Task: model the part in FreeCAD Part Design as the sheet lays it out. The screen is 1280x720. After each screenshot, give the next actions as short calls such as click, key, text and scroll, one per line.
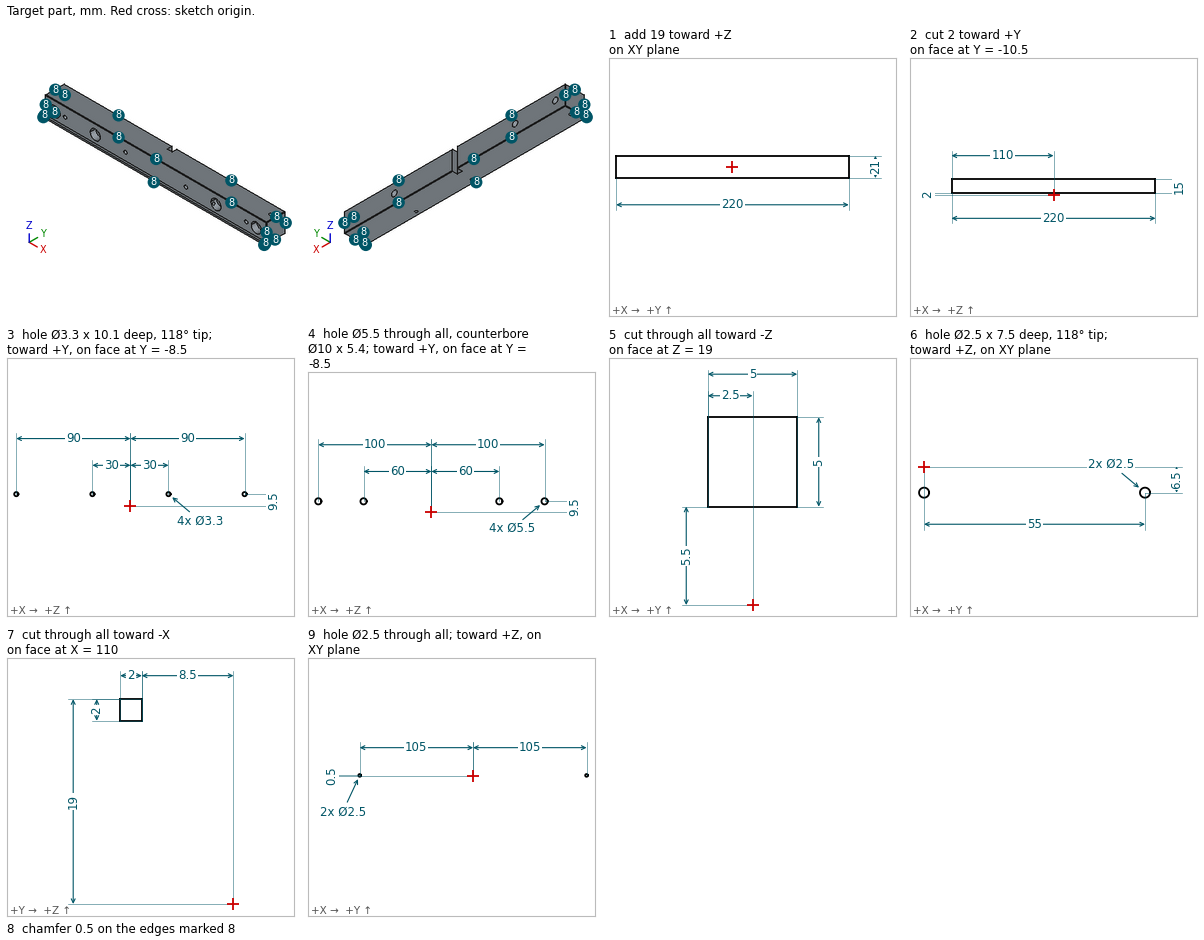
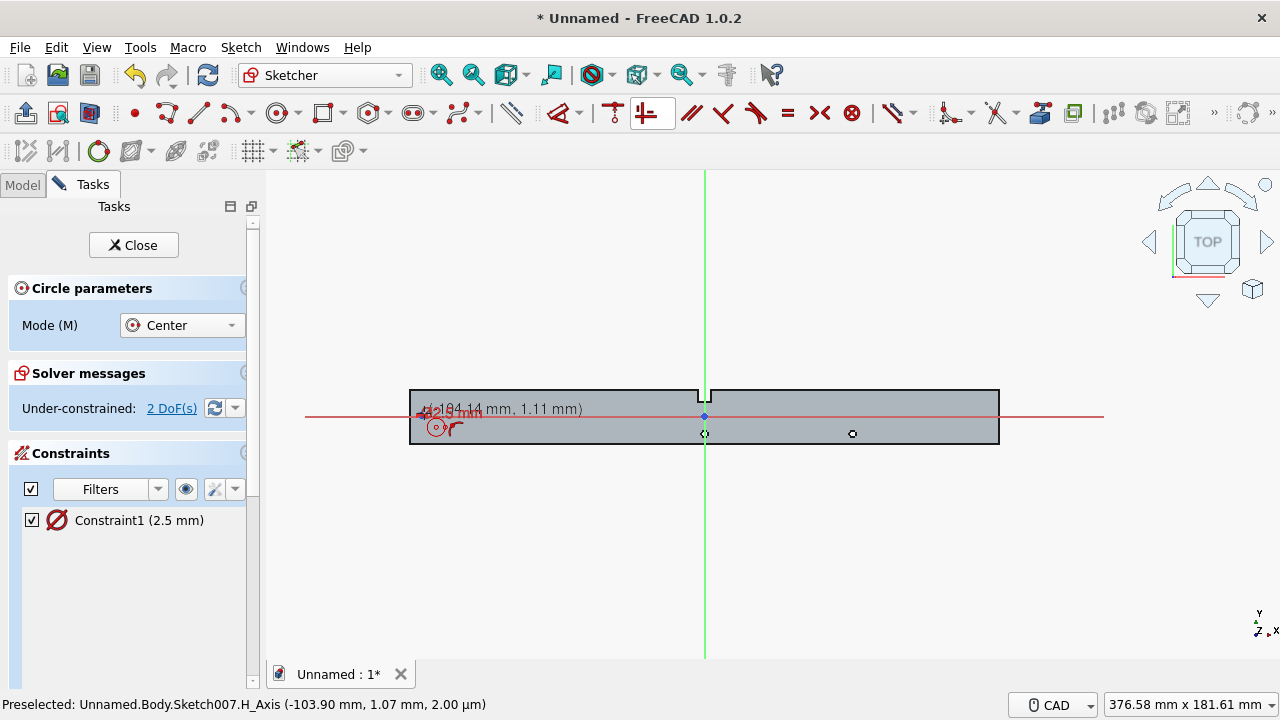
scroll(987, 415, up, 13)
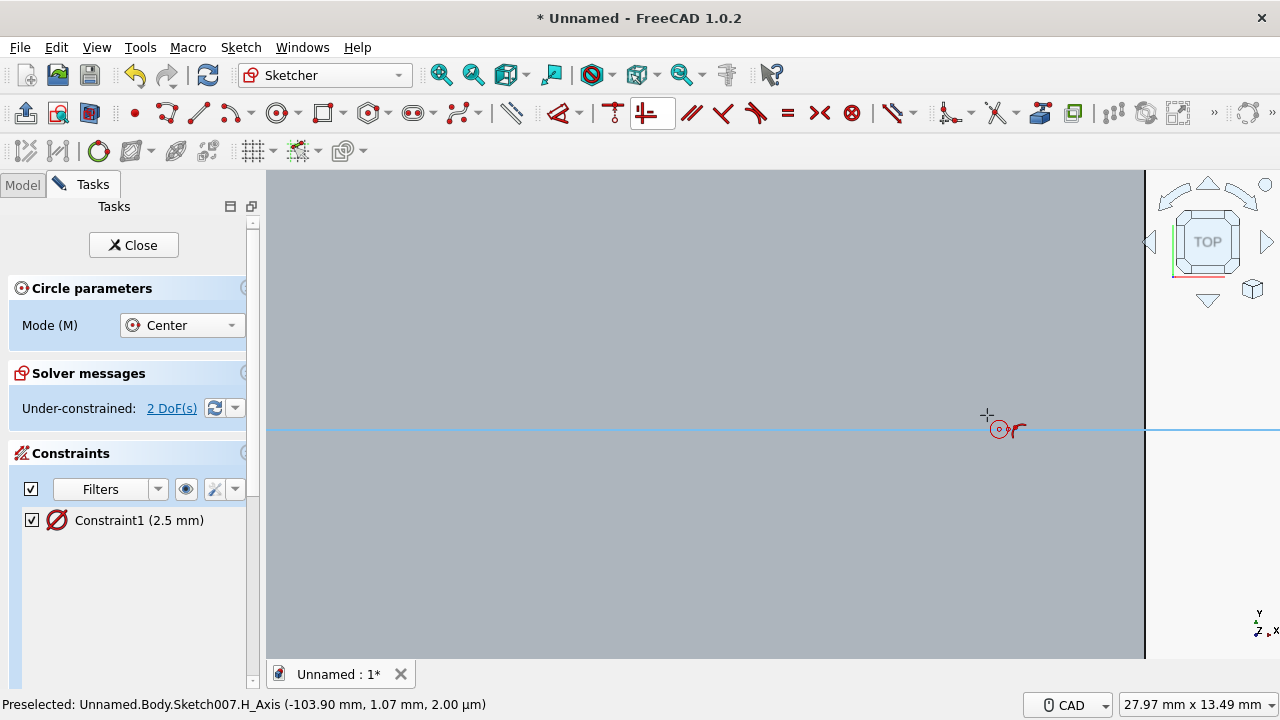
click(982, 412)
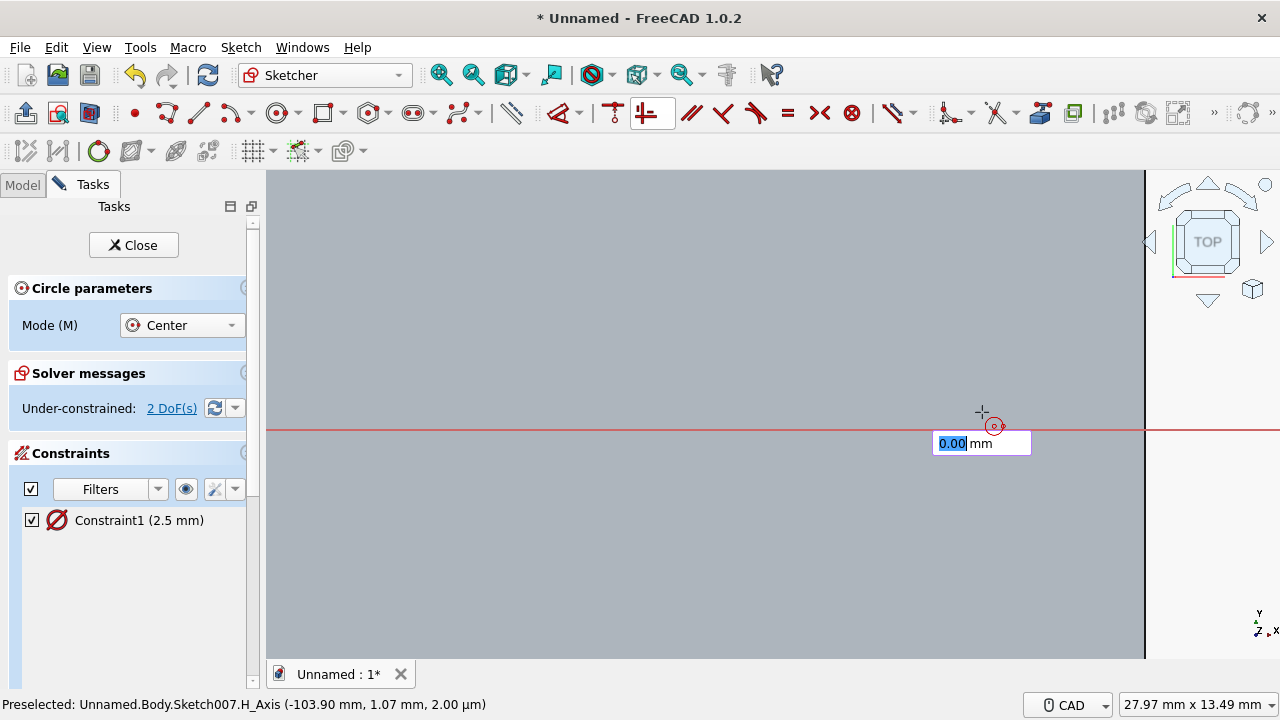
scroll(988, 415, down, 13)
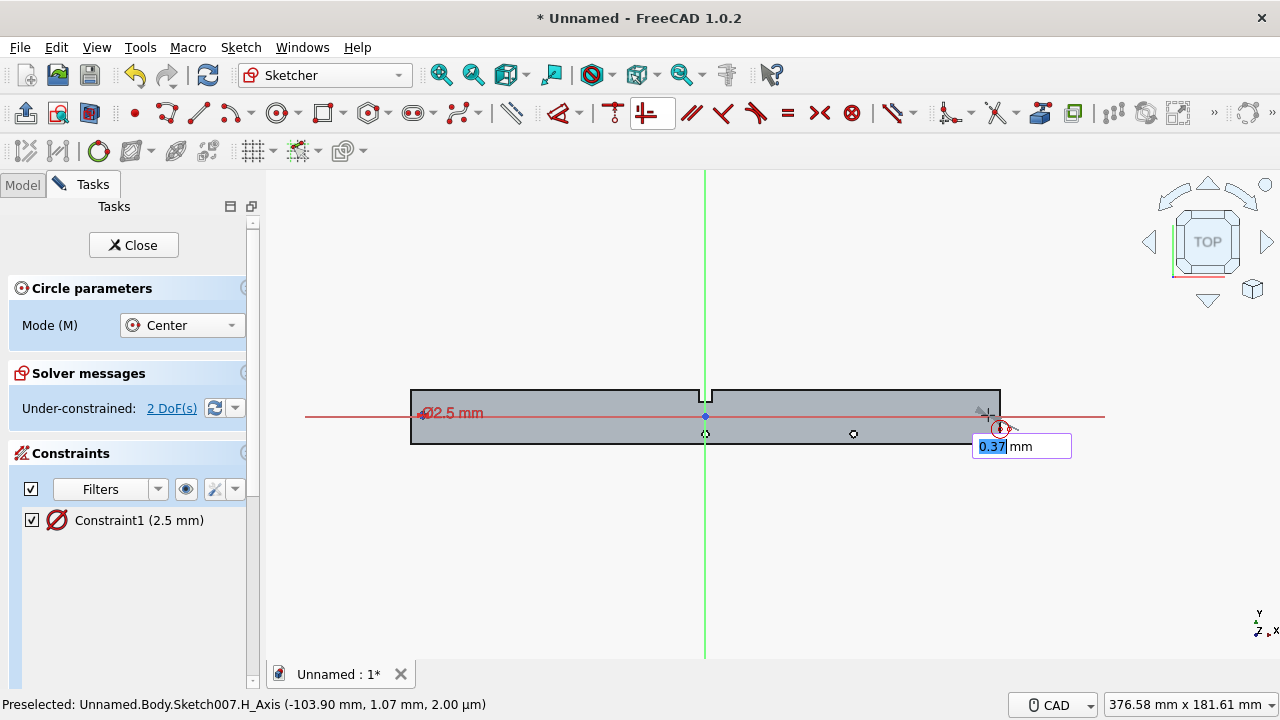
scroll(991, 413, up, 8)
move(986, 410)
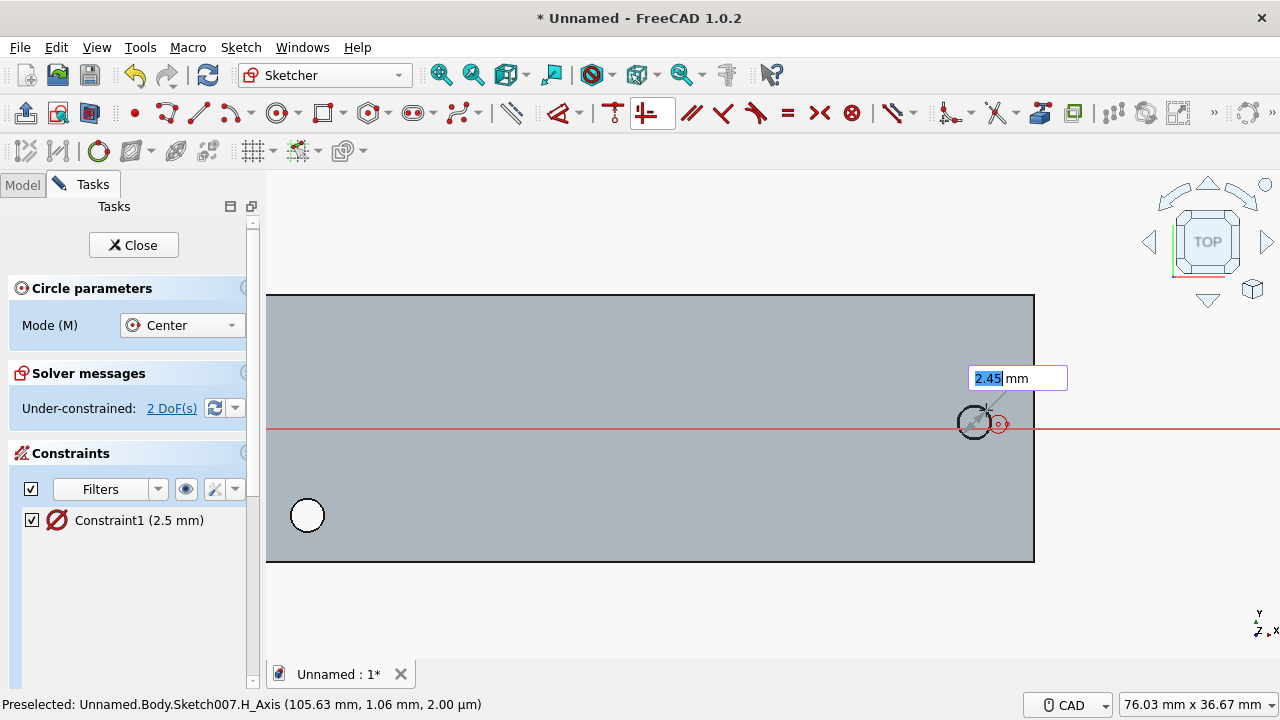
text(2.5)
key(Return)
key(Escape)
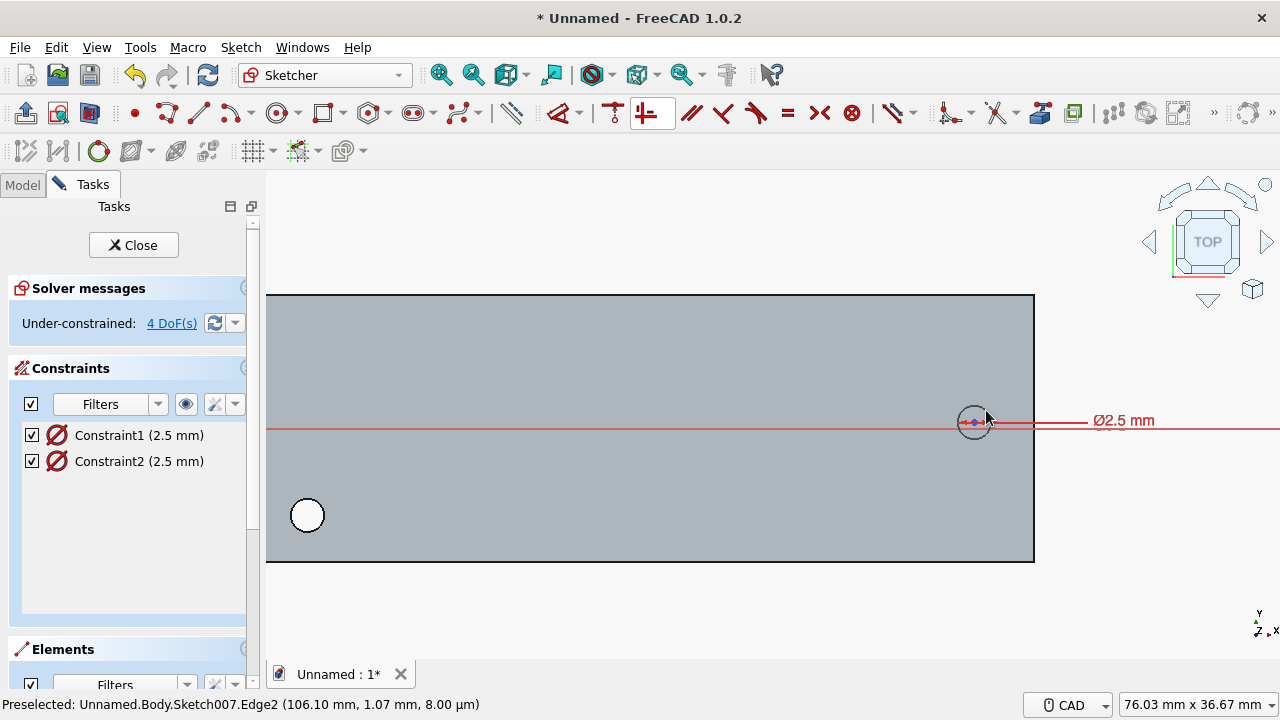
scroll(990, 413, down, 8)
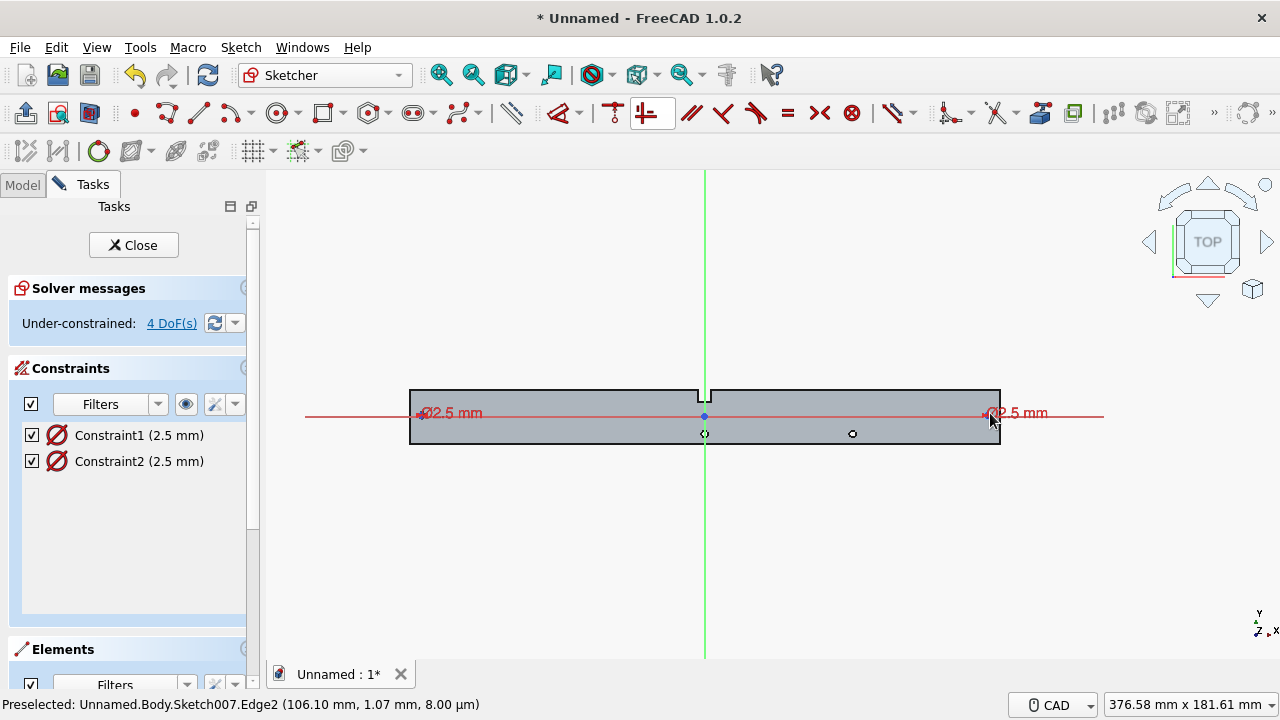
click(422, 415)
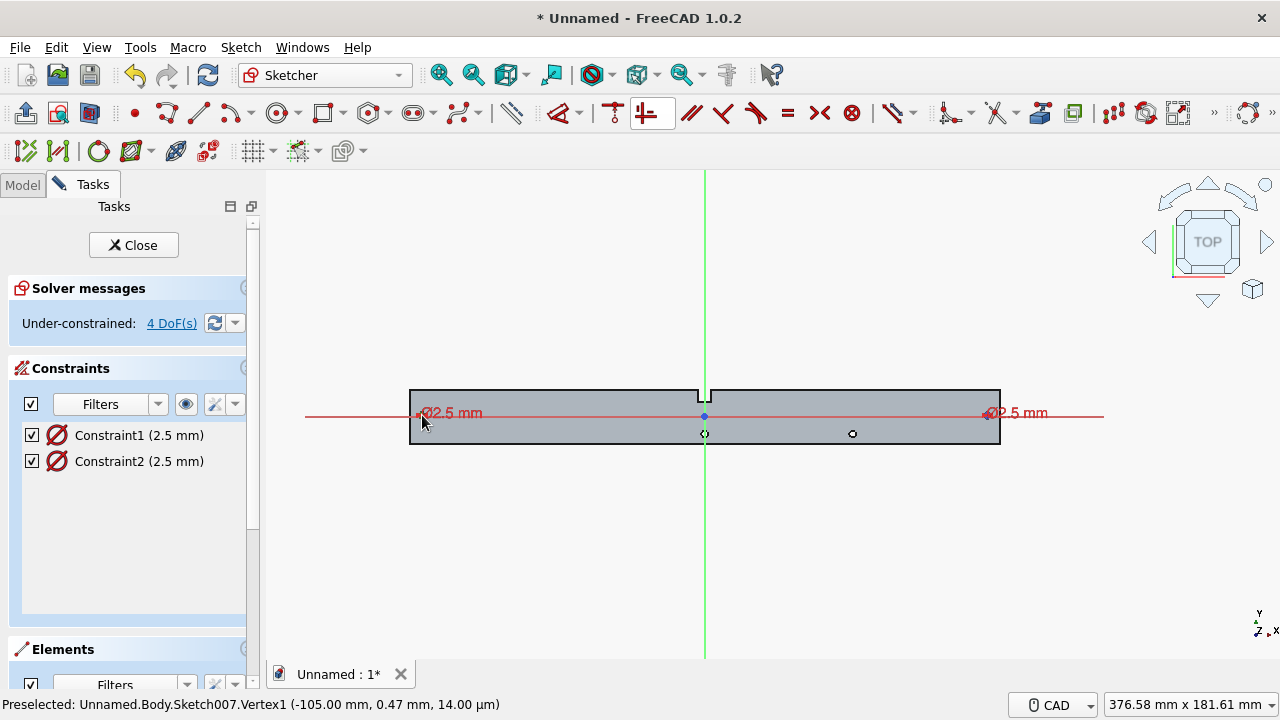
click(987, 415)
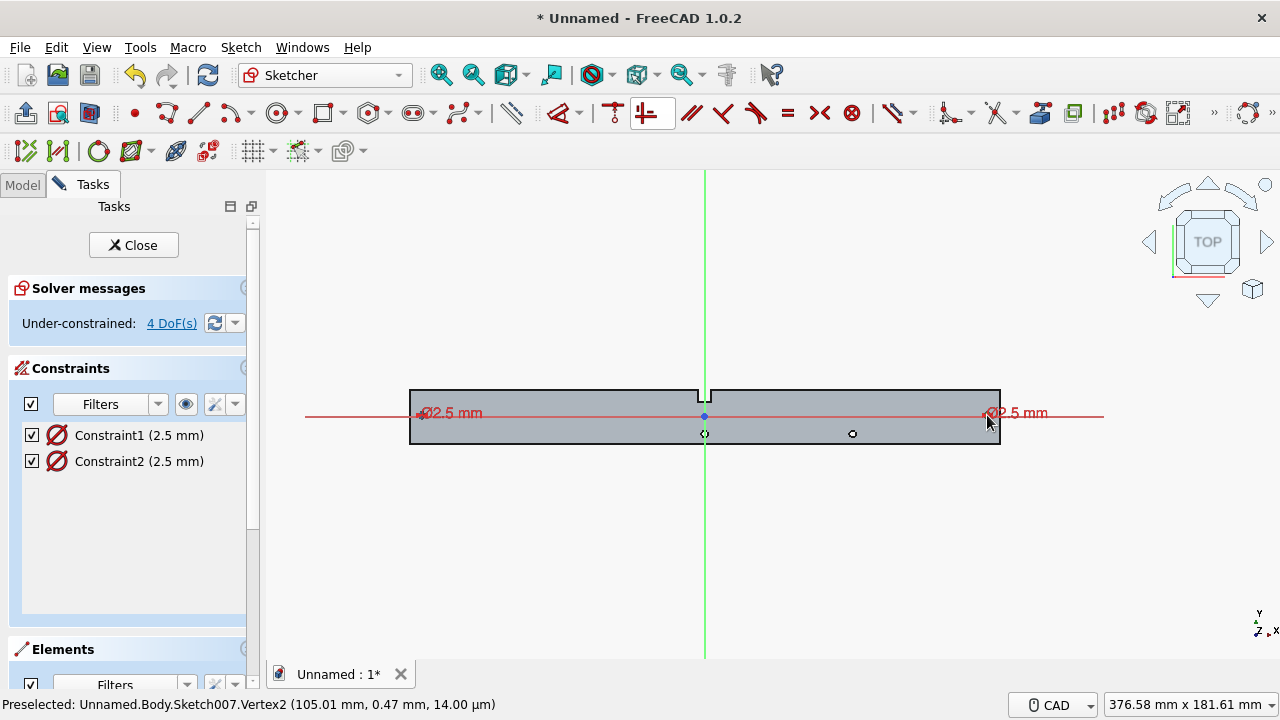
click(670, 114)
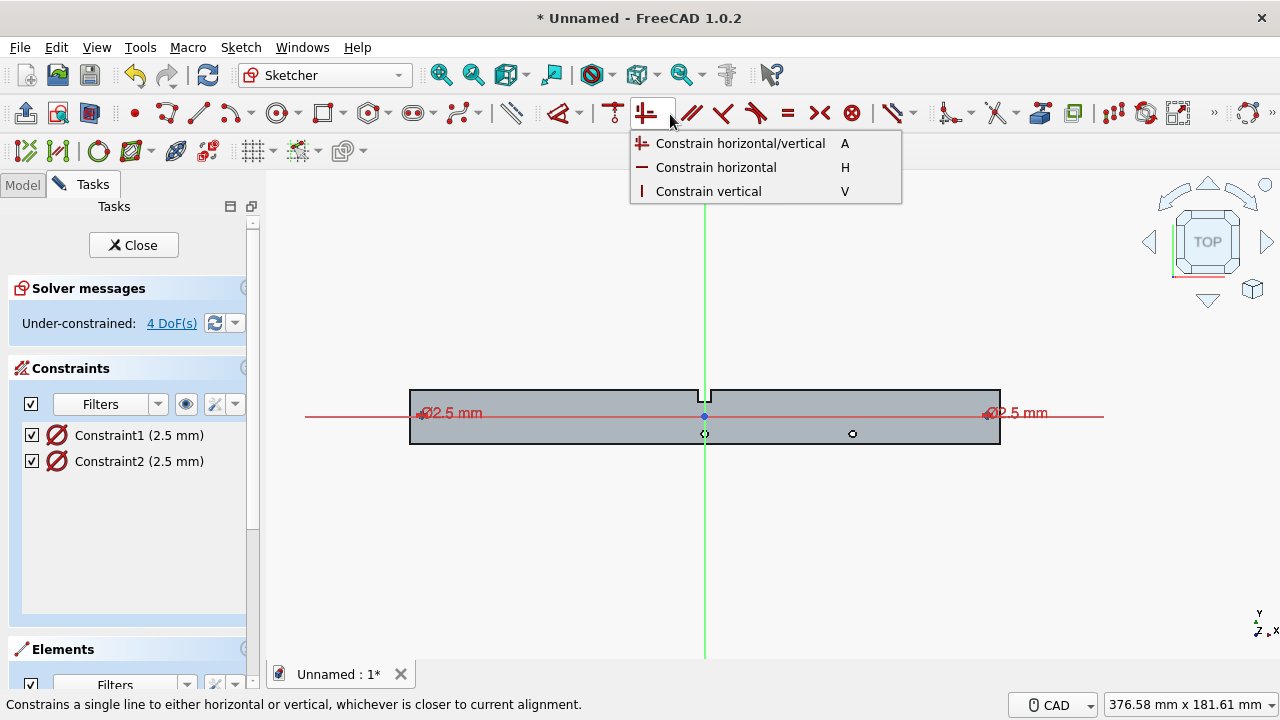
click(766, 167)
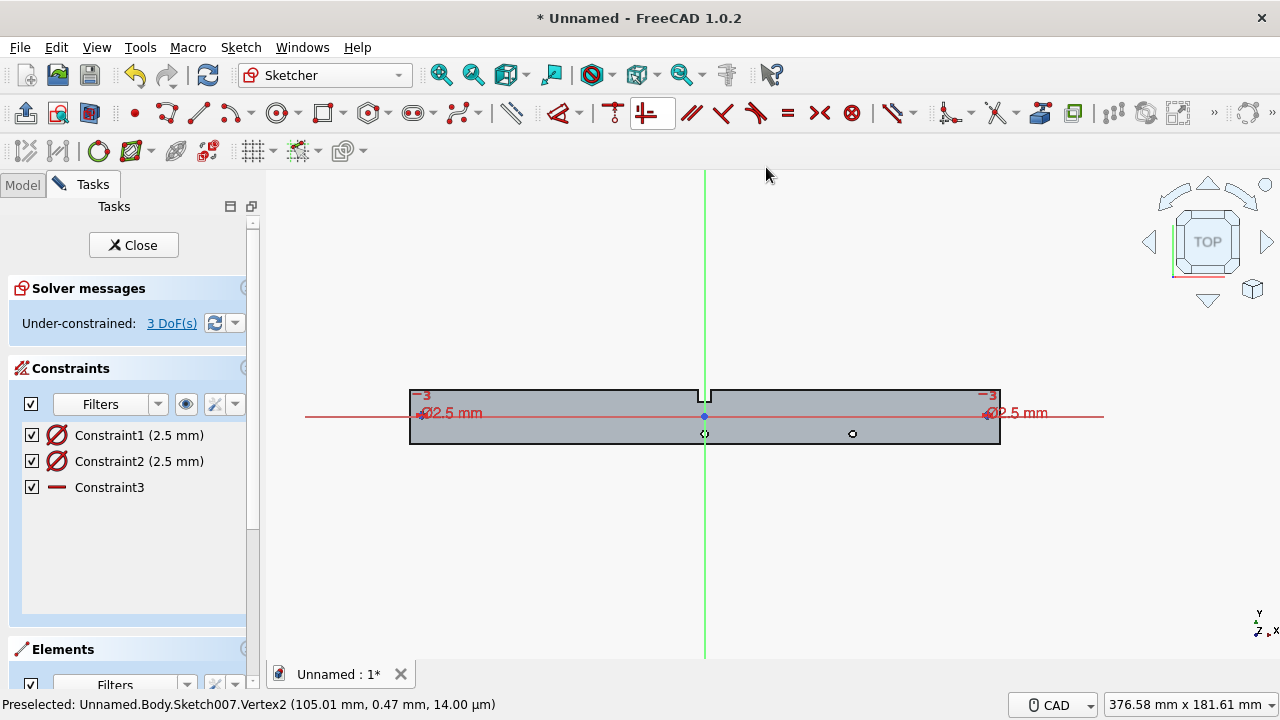
click(558, 114)